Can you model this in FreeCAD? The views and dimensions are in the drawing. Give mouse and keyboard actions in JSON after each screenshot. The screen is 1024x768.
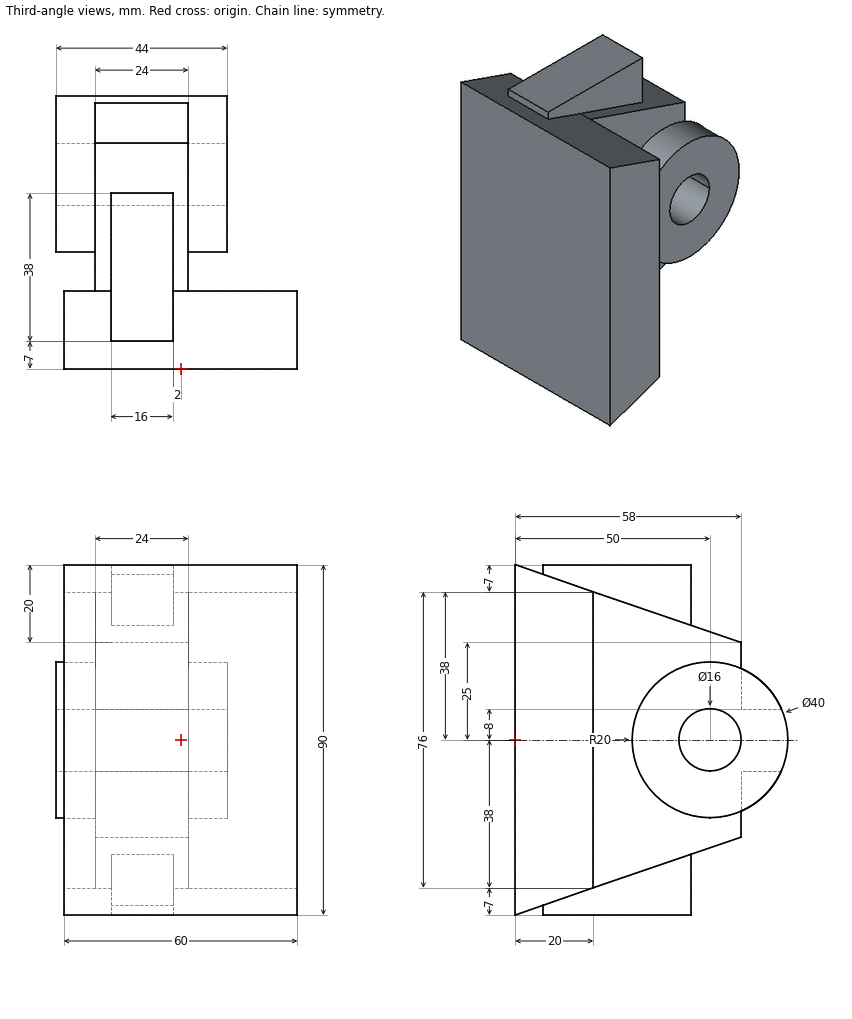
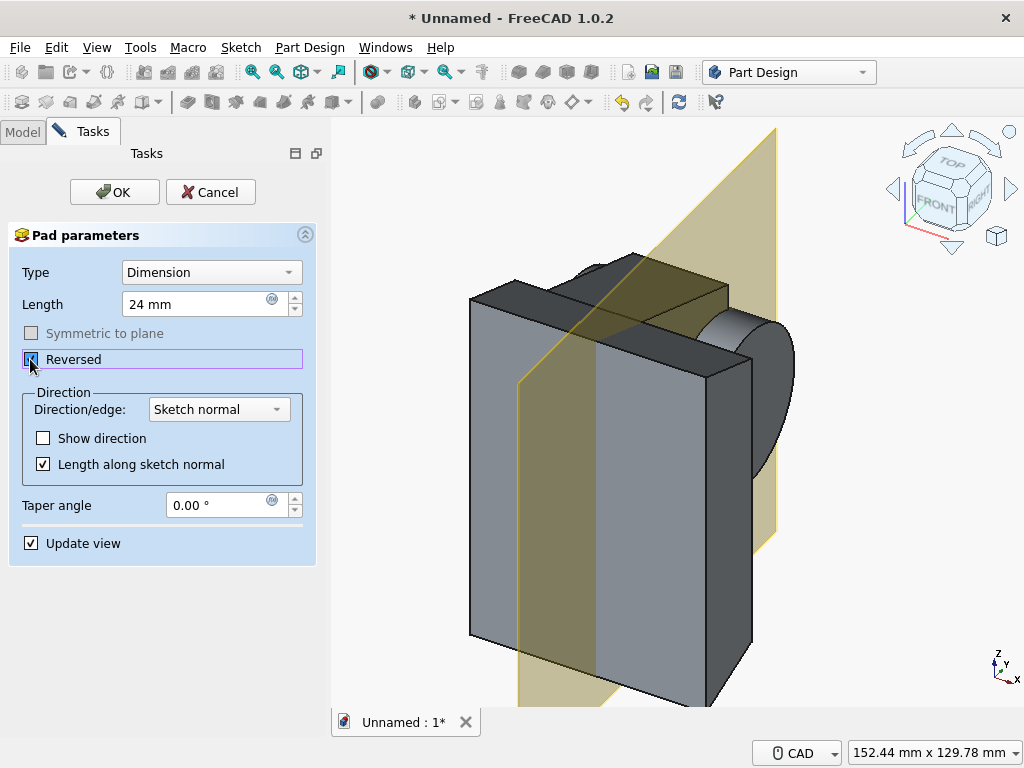
{"action": "left_click", "coordinate": [115, 192]}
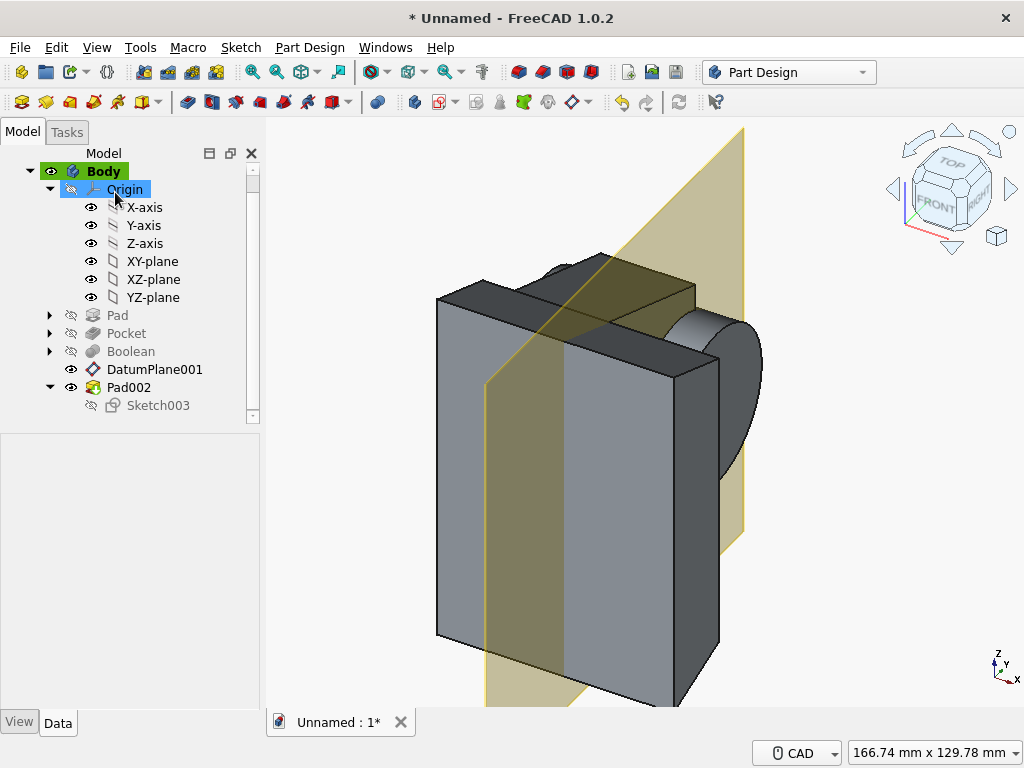
{"action": "left_click", "coordinate": [116, 369]}
{"action": "key", "text": "space"}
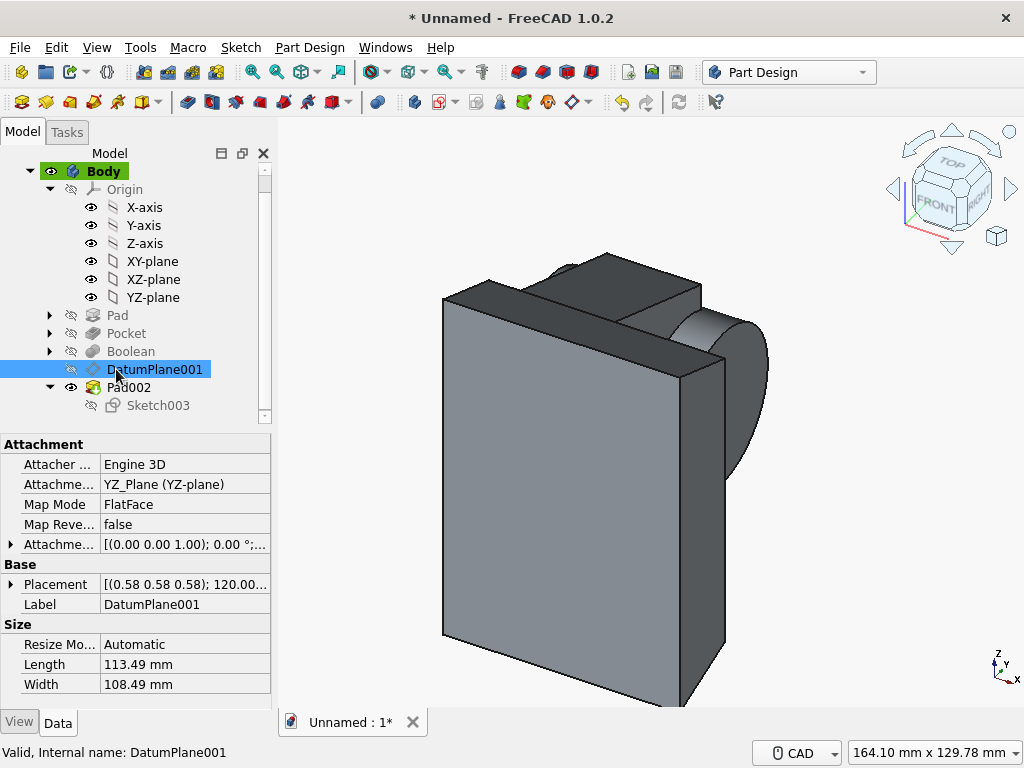
{"action": "left_click", "coordinate": [254, 72]}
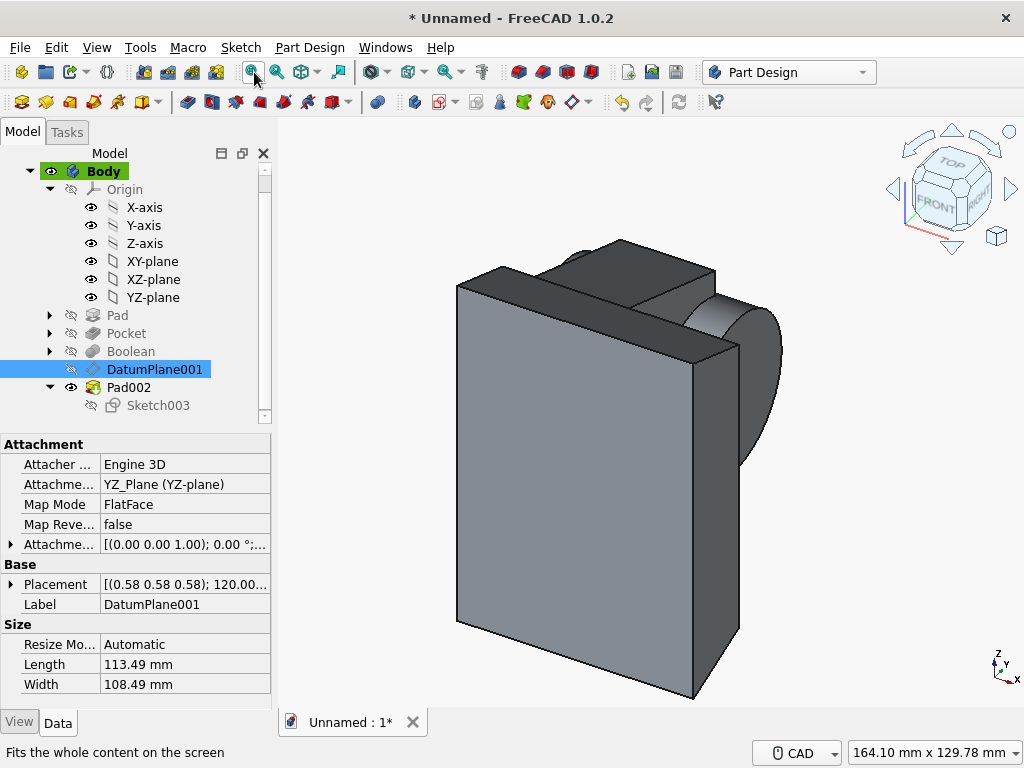
{"action": "key", "text": "0"}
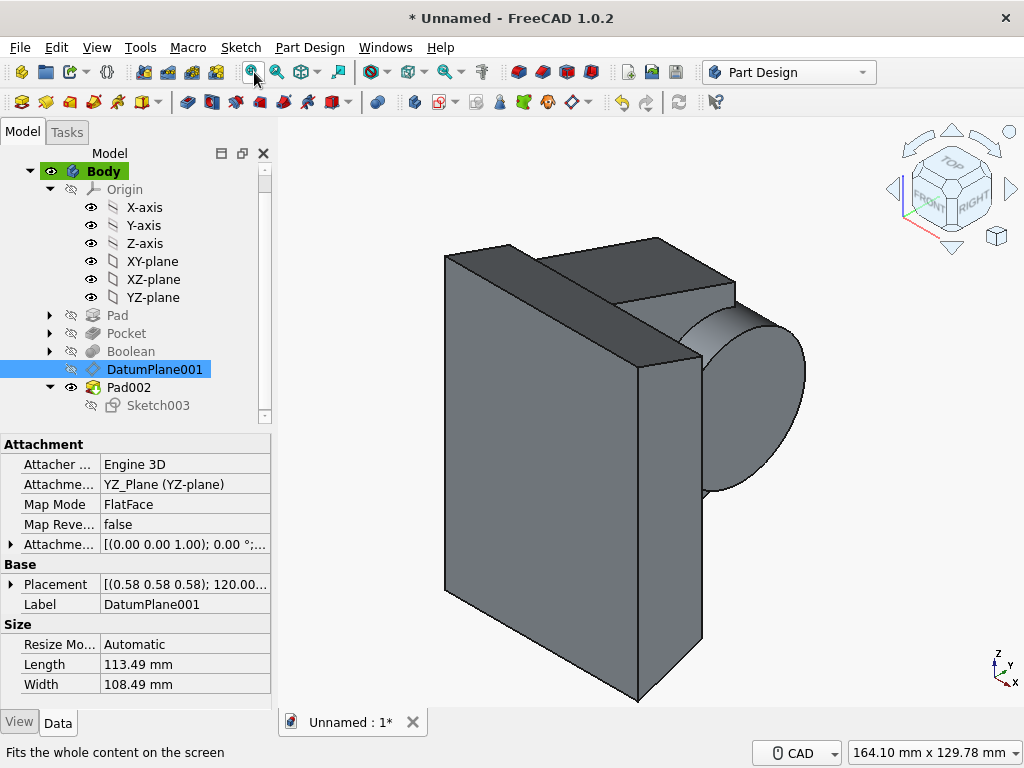
{"action": "key", "text": "3"}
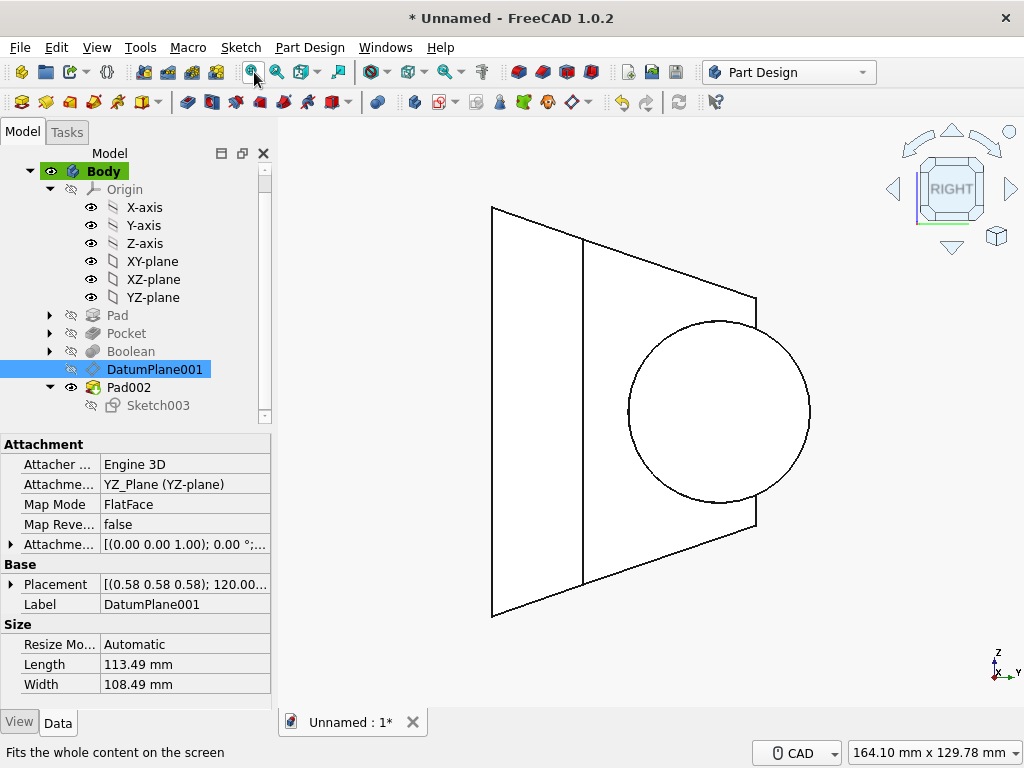
{"action": "left_click", "coordinate": [620, 312]}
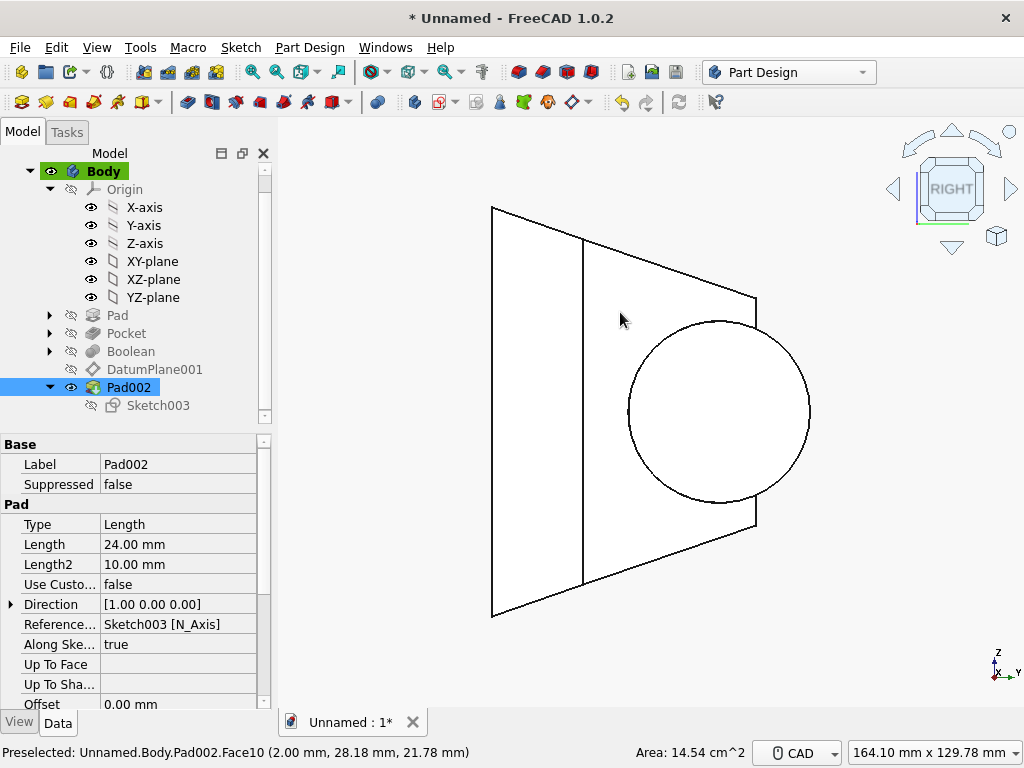
{"action": "left_click", "coordinate": [440, 102]}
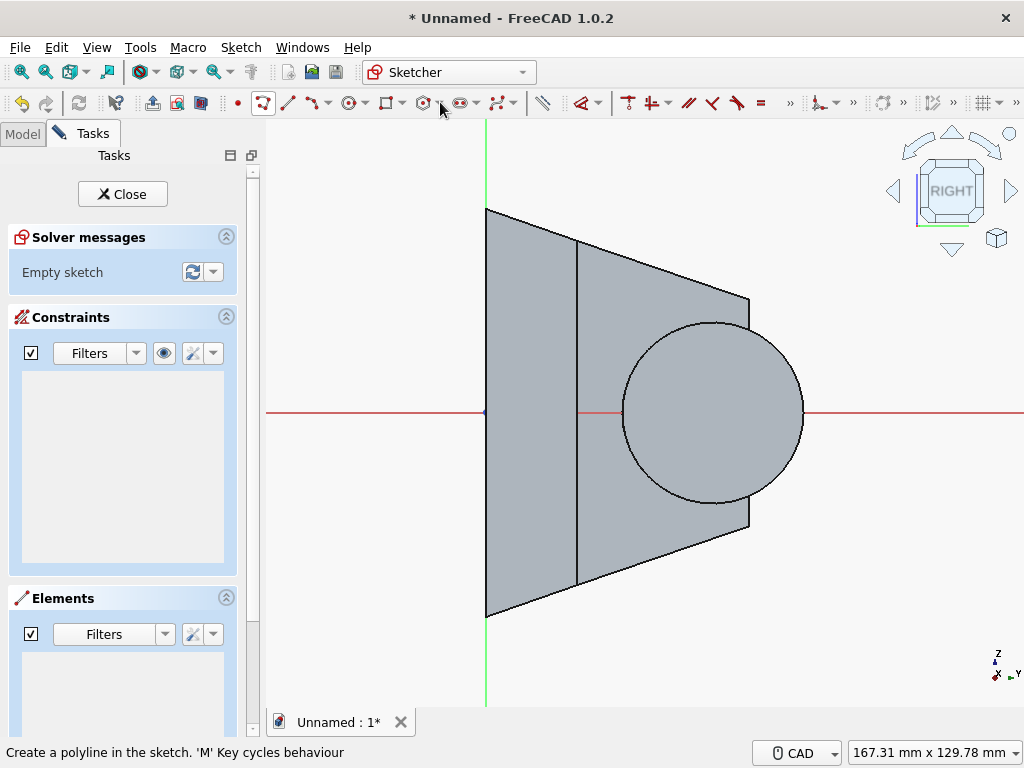
{"action": "key", "text": "q s"}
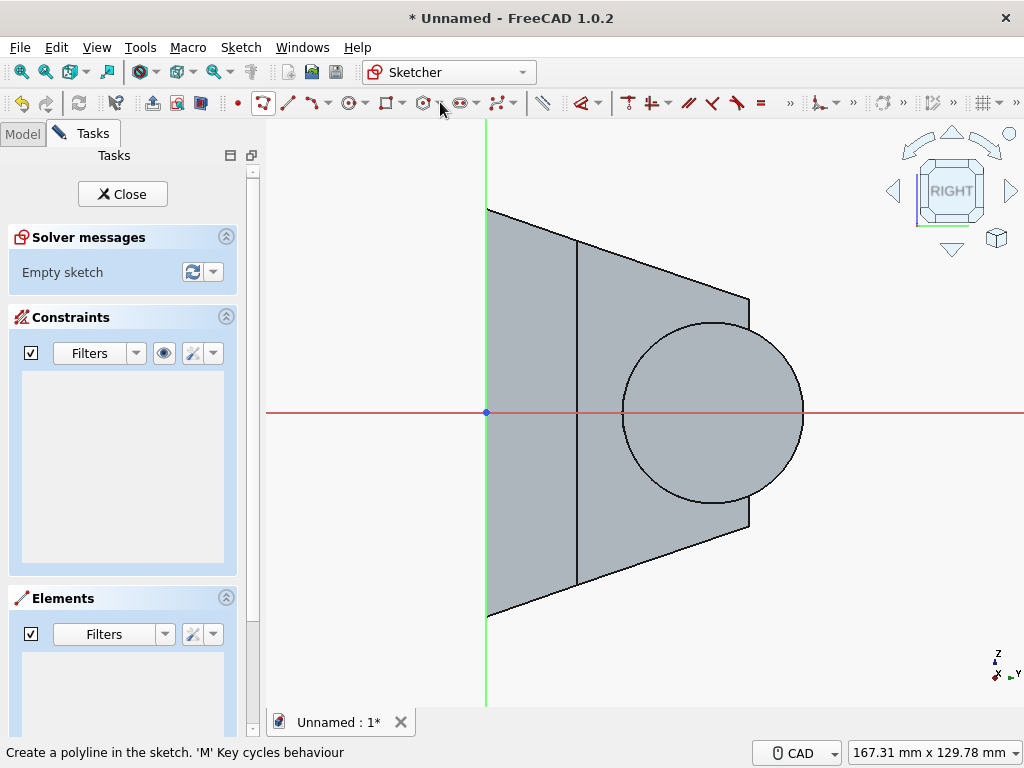
{"action": "scroll", "coordinate": [803, 344], "scroll_direction": "up", "scroll_amount": 10}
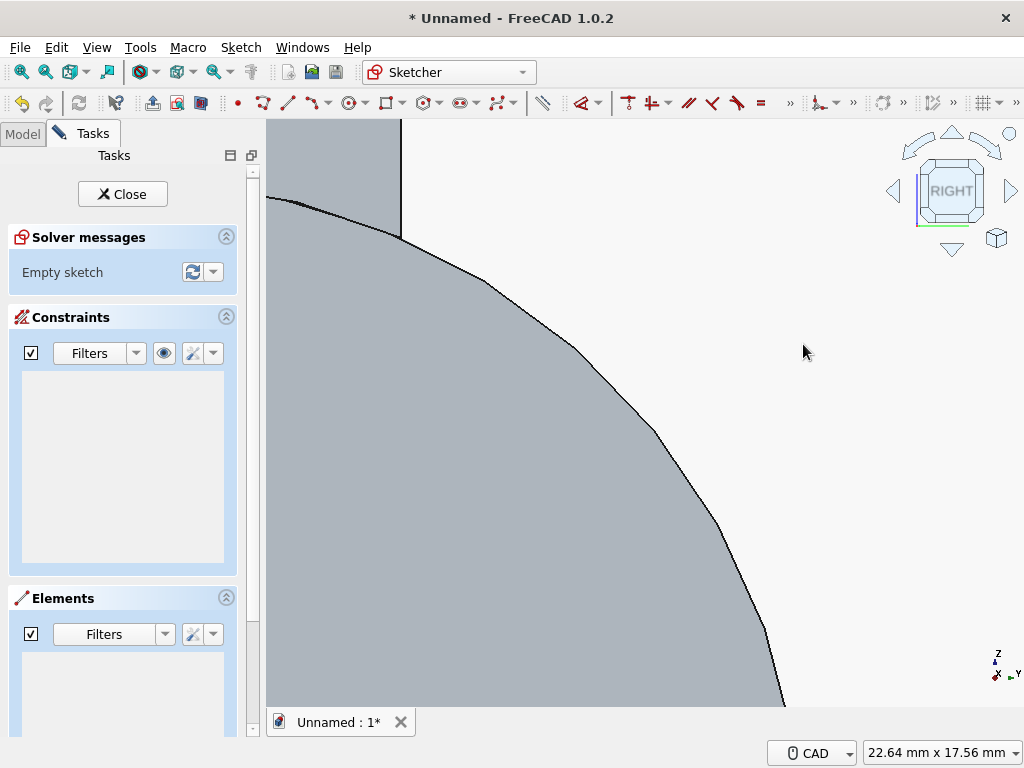
{"action": "left_click", "coordinate": [264, 104]}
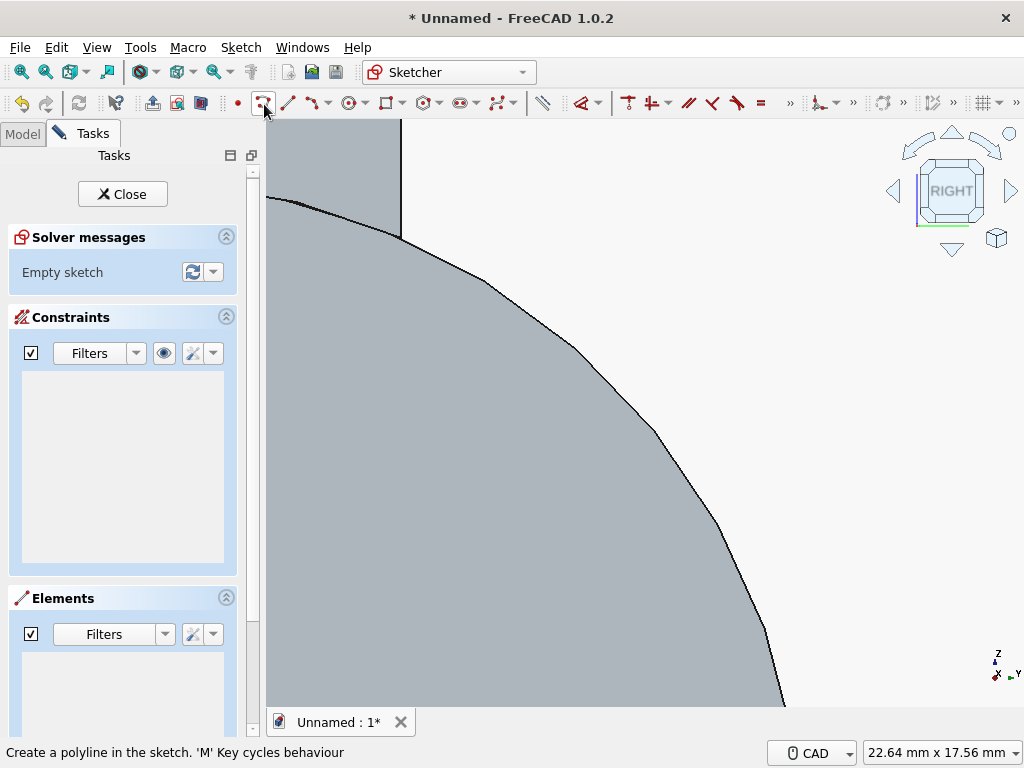
{"action": "left_click", "coordinate": [401, 238]}
{"action": "left_click", "coordinate": [401, 584]}
{"action": "left_click", "coordinate": [747, 584]}
{"action": "right_click", "coordinate": [747, 584]}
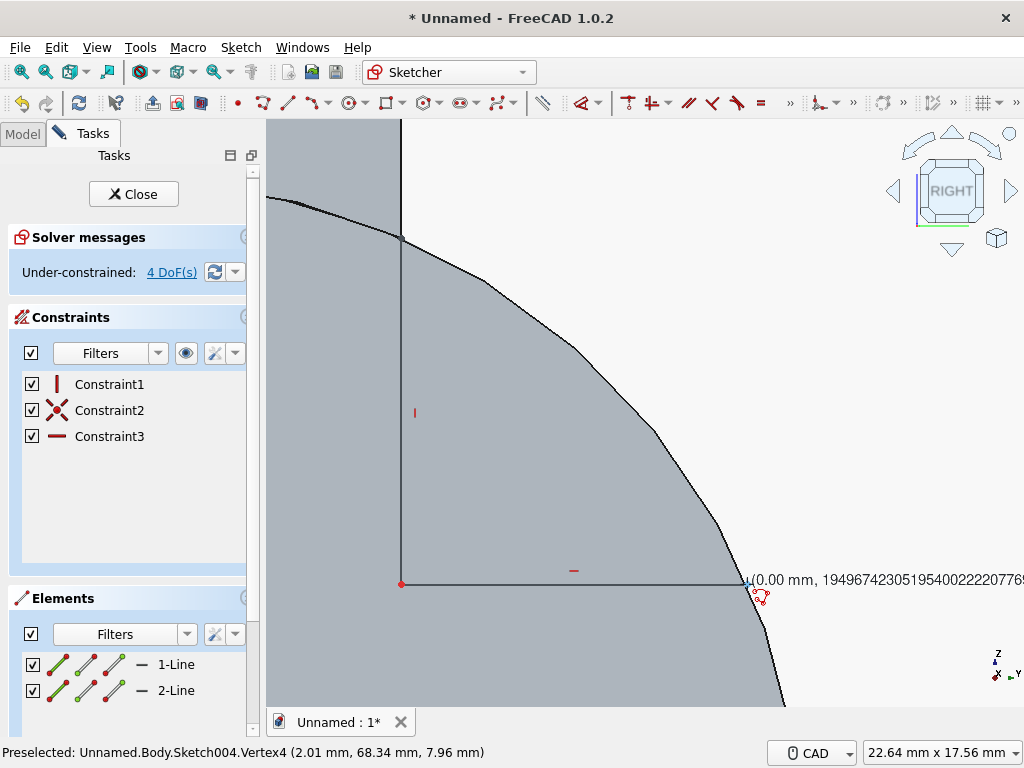
{"action": "left_click", "coordinate": [312, 104]}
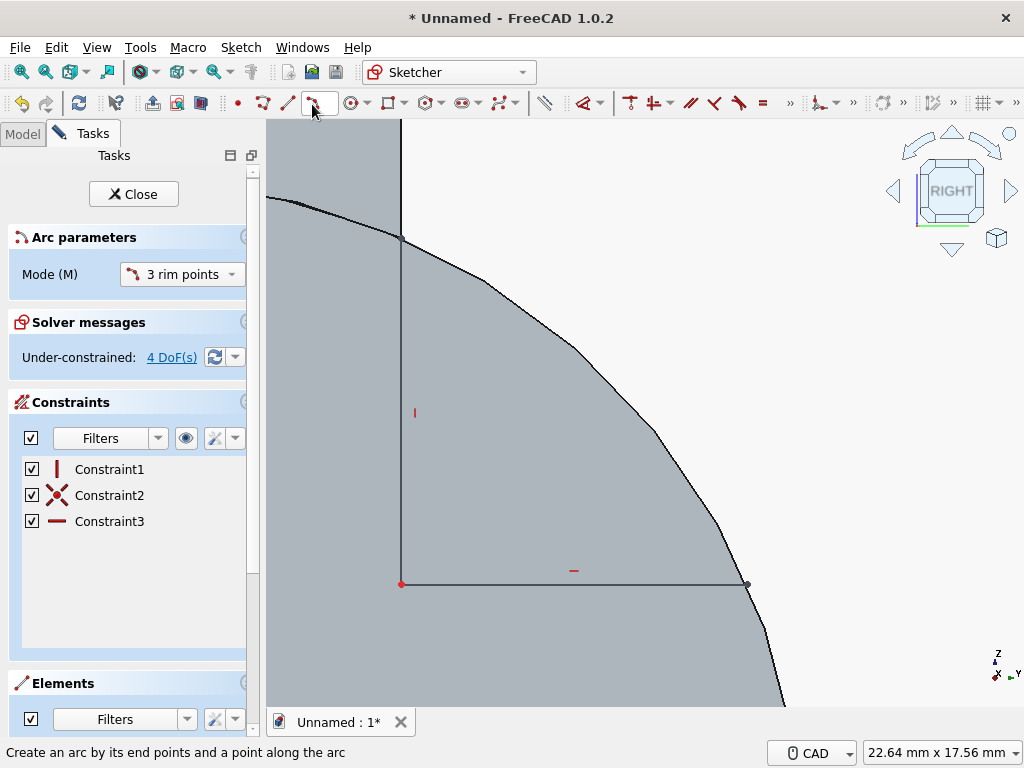
{"action": "left_click", "coordinate": [747, 585]}
{"action": "left_click", "coordinate": [401, 239]}
{"action": "left_click", "coordinate": [607, 378]}
{"action": "key", "text": "Escape"}